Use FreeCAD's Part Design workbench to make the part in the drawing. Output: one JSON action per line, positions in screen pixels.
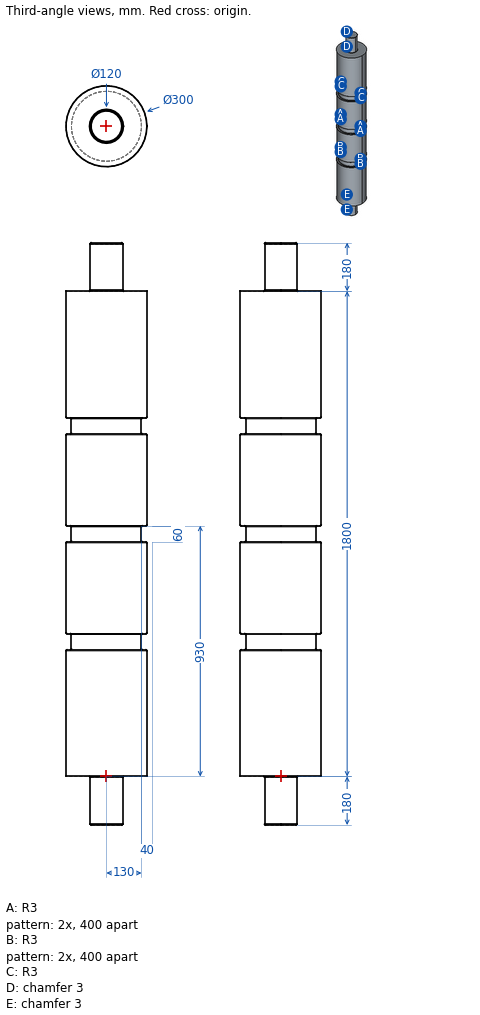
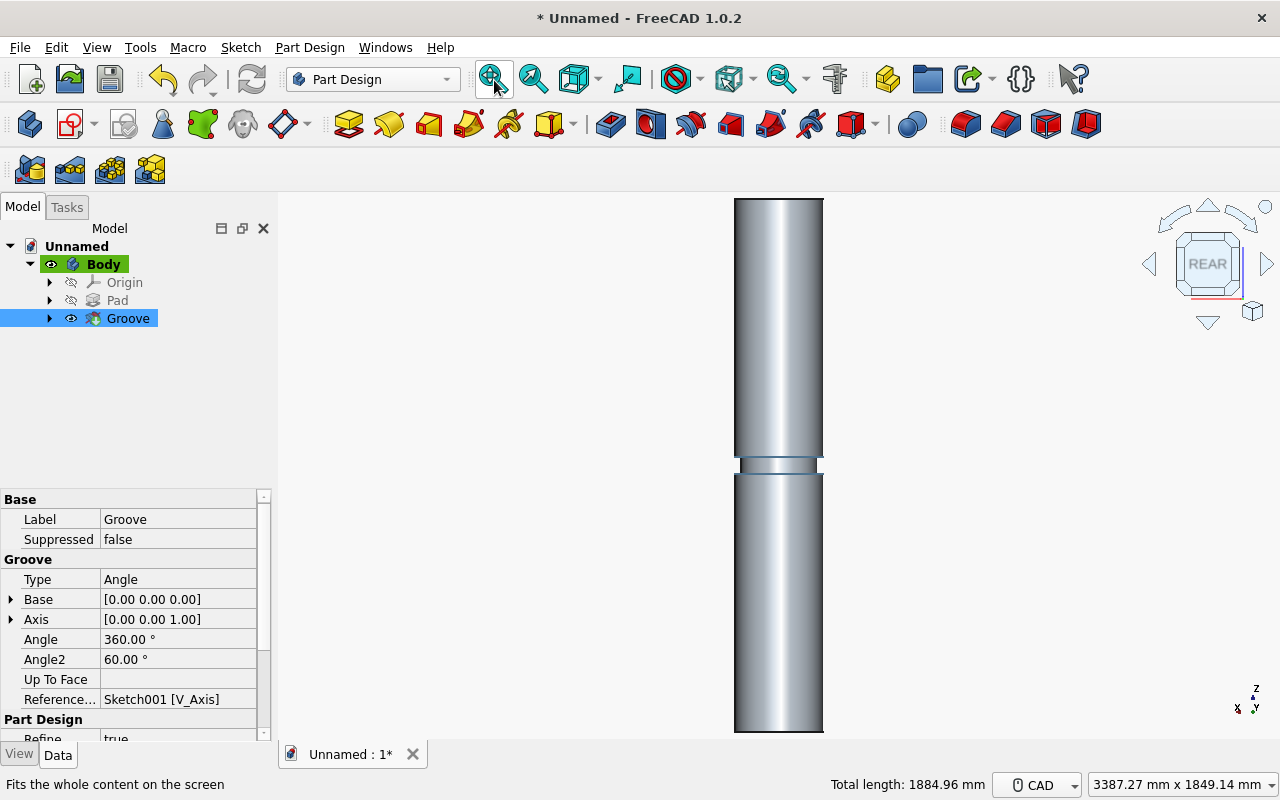
{"action": "key", "text": "6"}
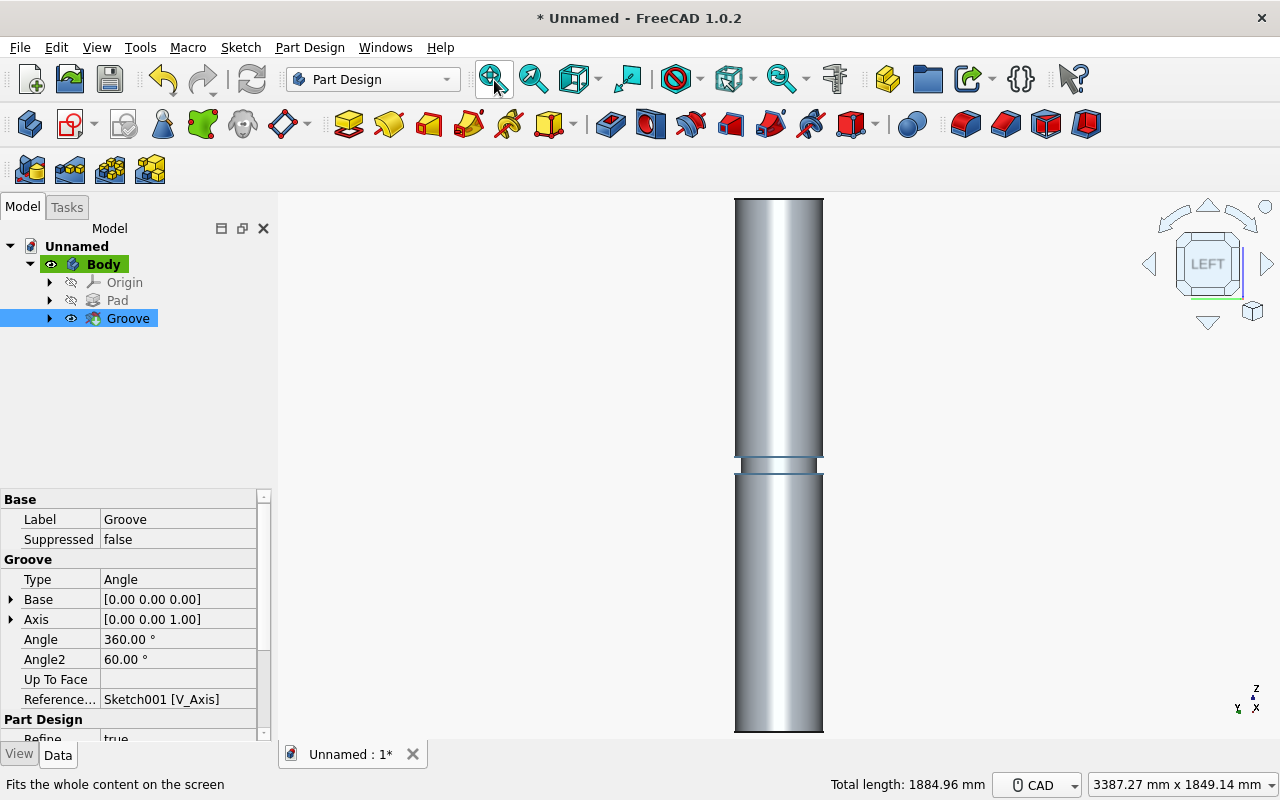
{"action": "key", "text": "v 3"}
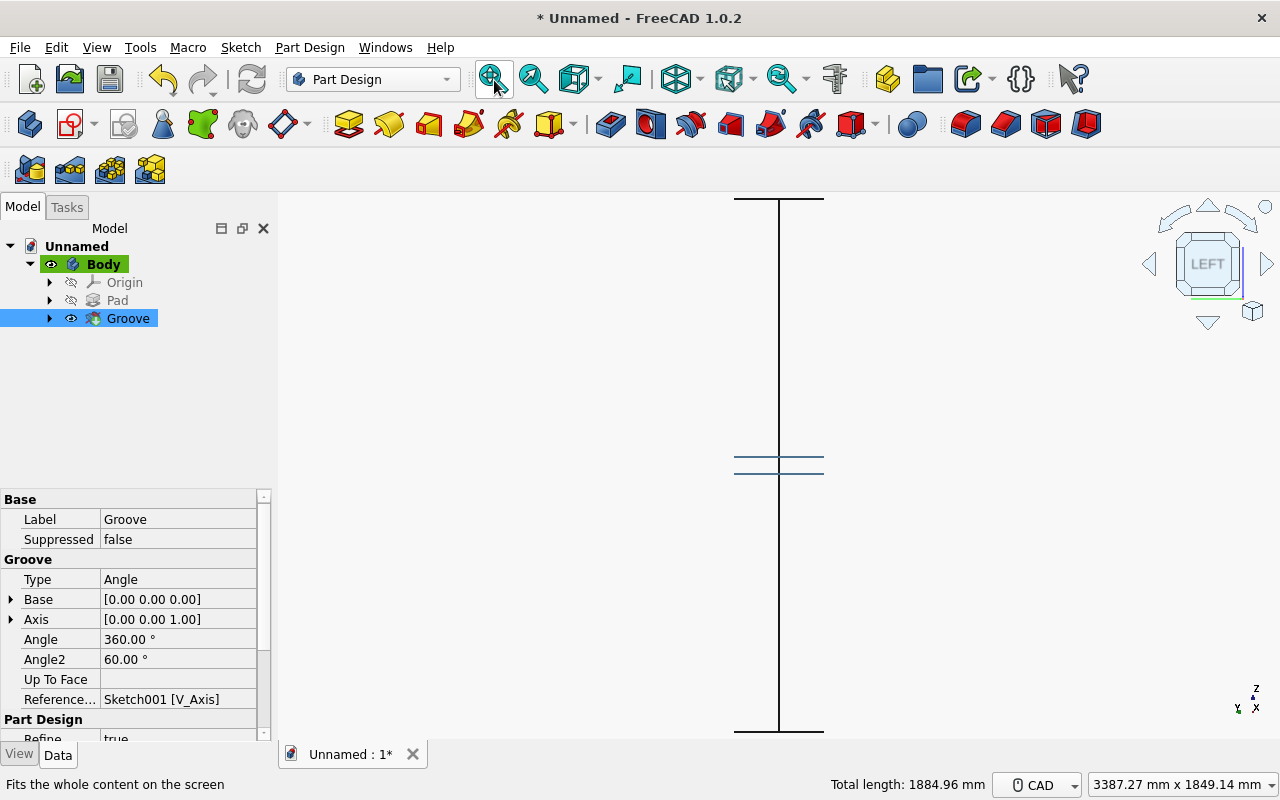
{"action": "key", "text": "0"}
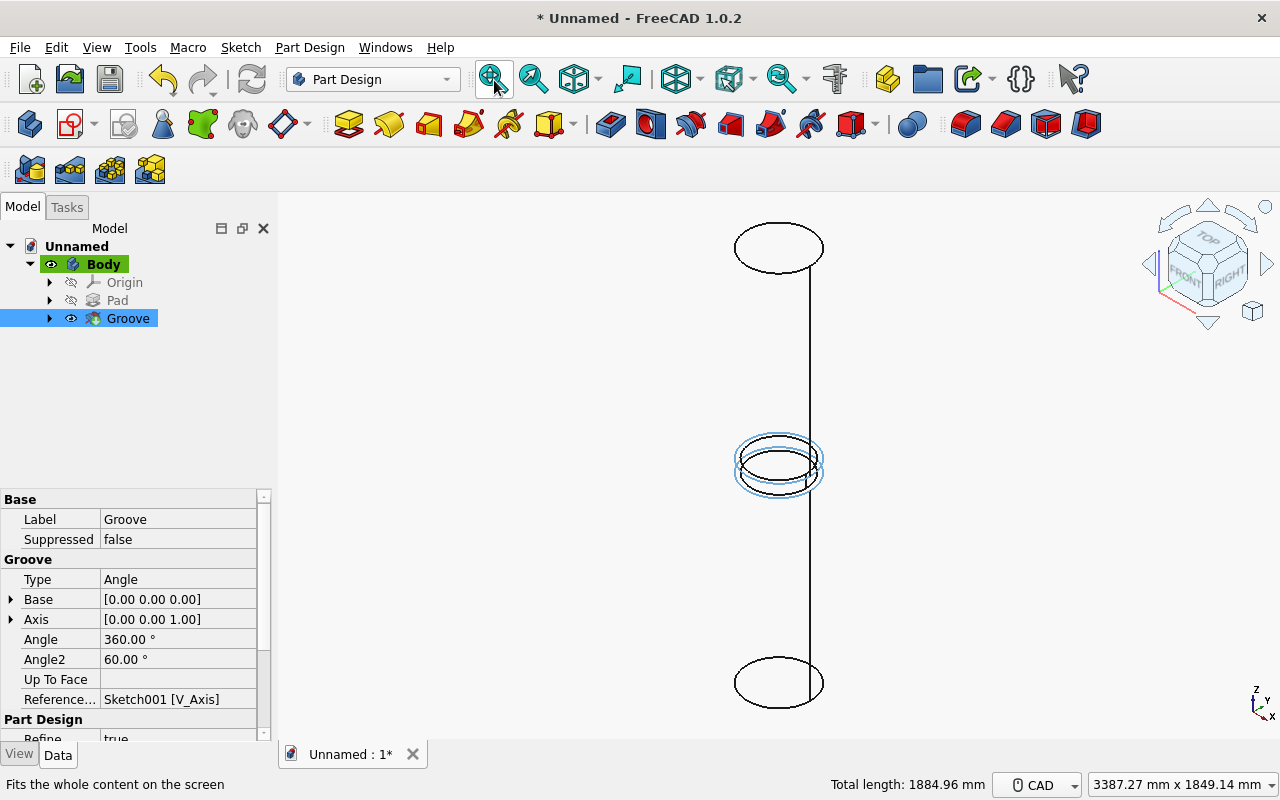
{"action": "left_click", "coordinate": [752, 442], "text": "ctrl"}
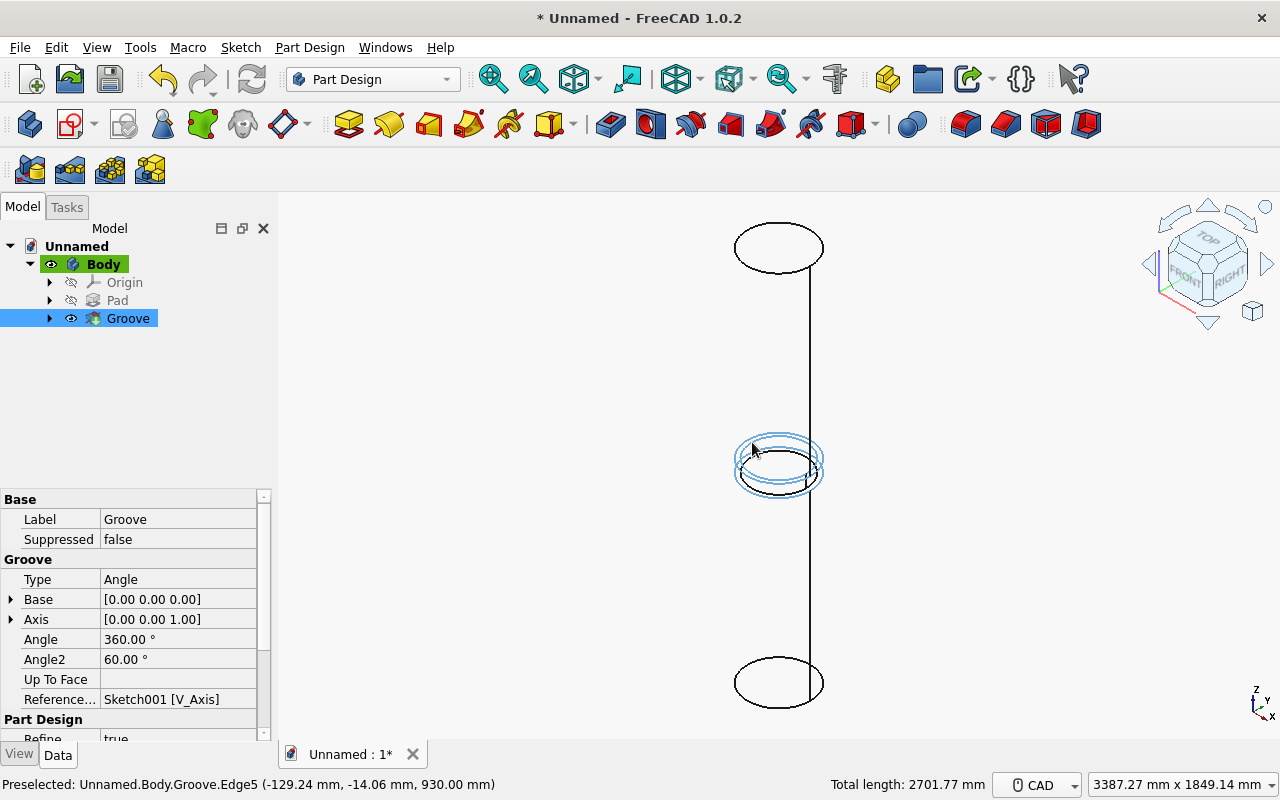
{"action": "left_click", "coordinate": [752, 456], "text": "ctrl"}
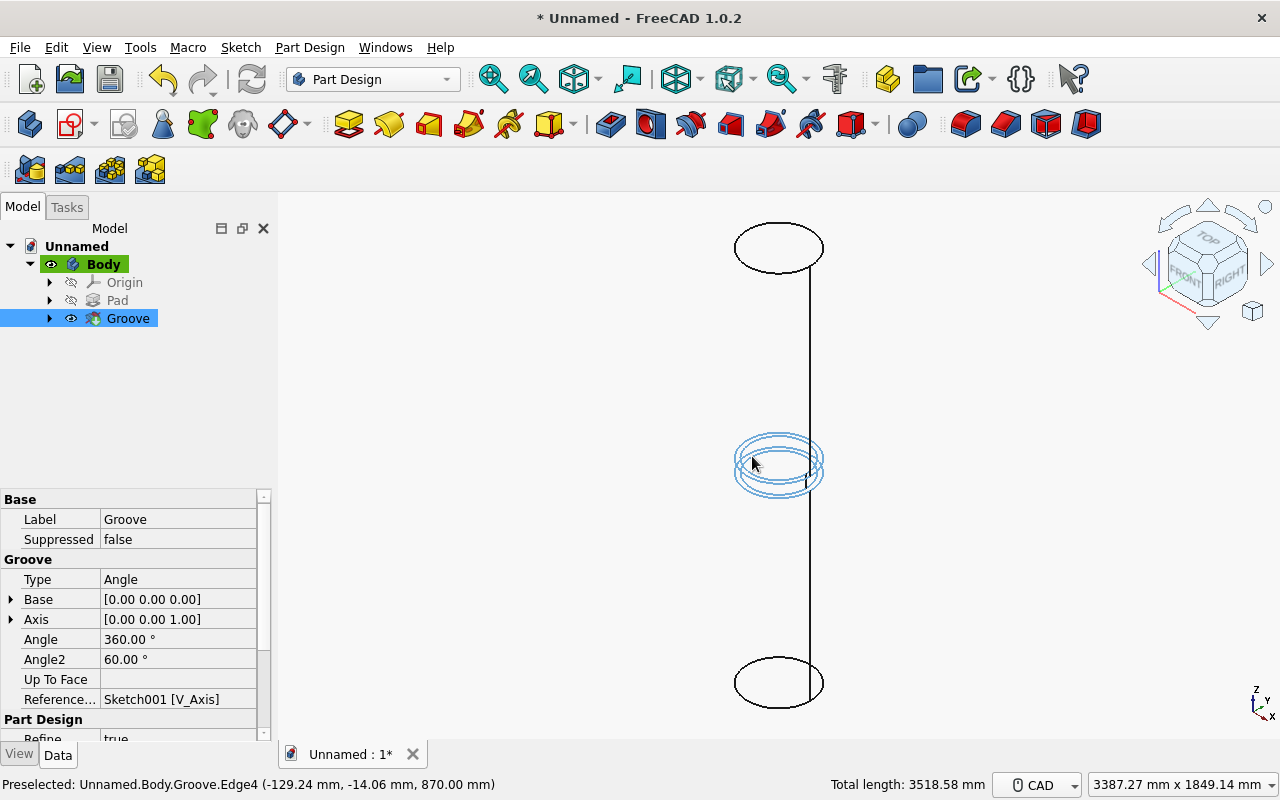
{"action": "key", "text": "v 1"}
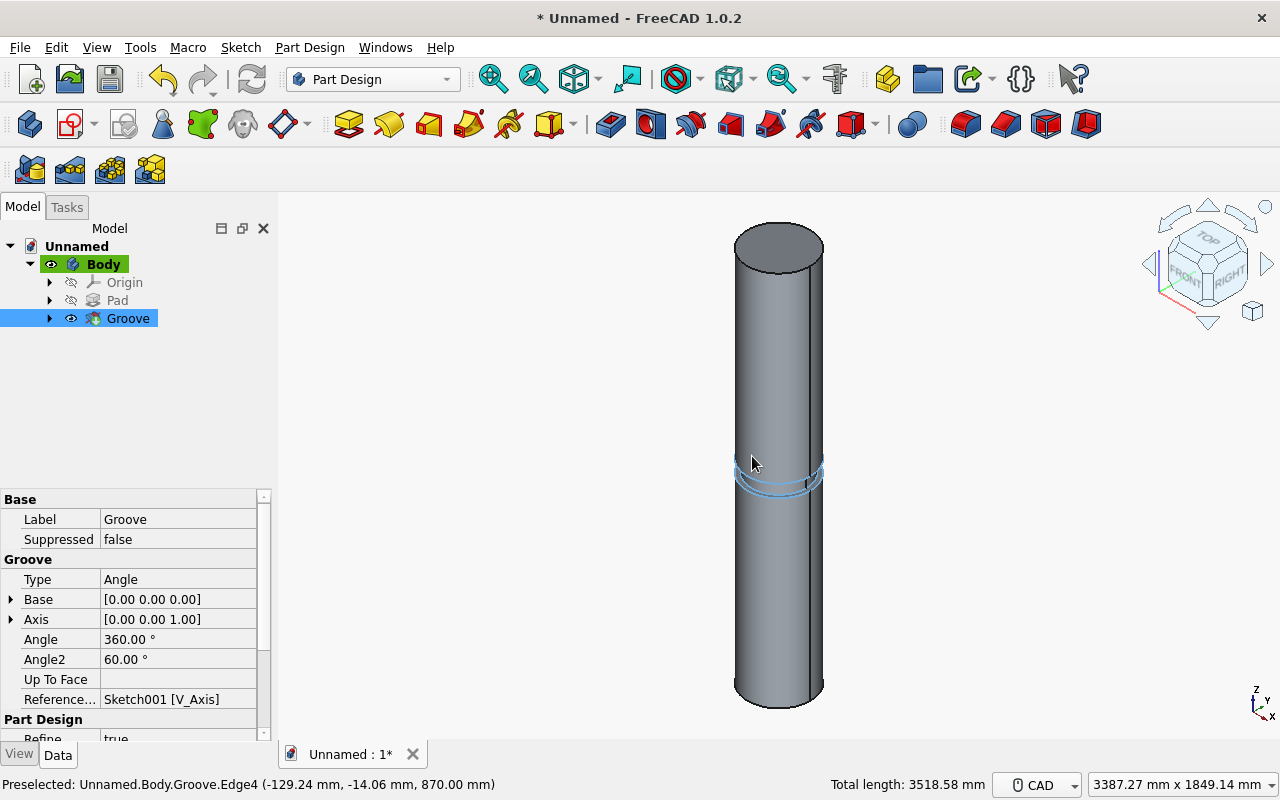
{"action": "left_click", "coordinate": [966, 124]}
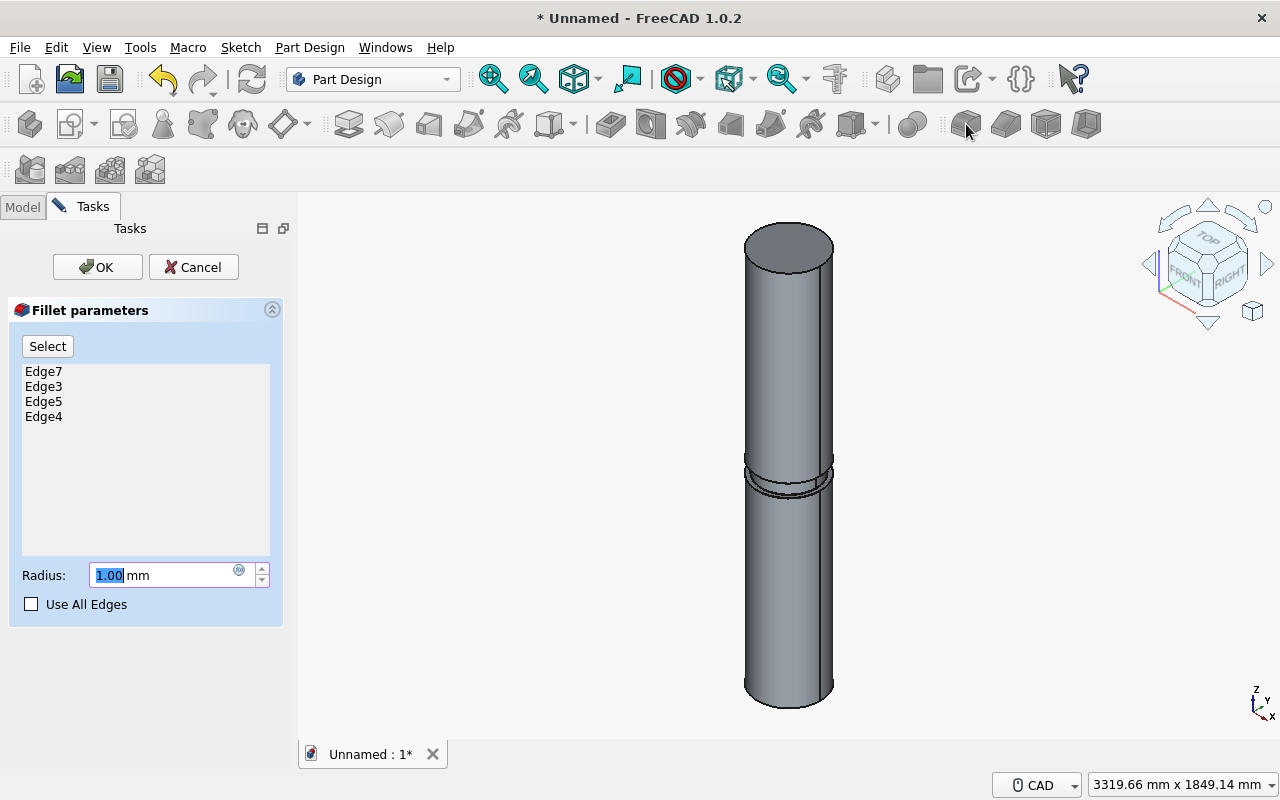
{"action": "type", "text": "3"}
{"action": "key", "text": "Tab"}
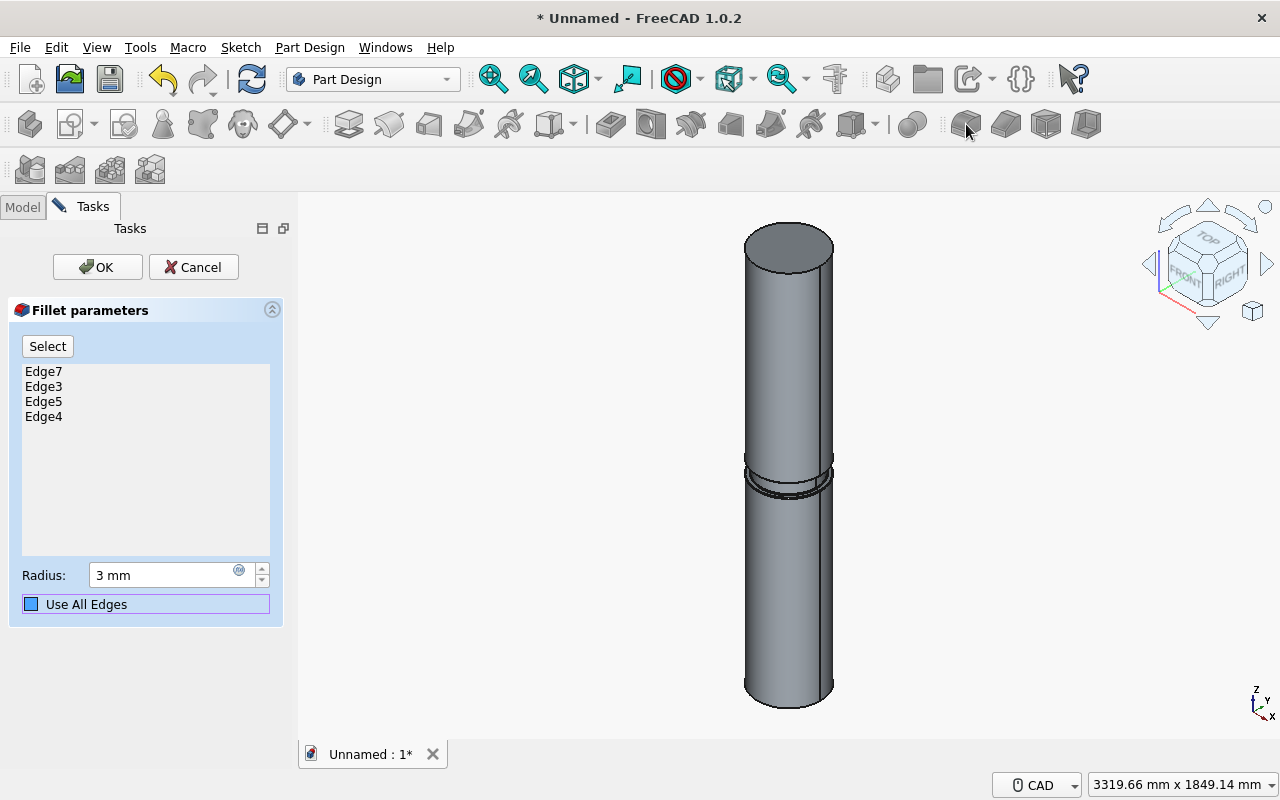
{"action": "left_click", "coordinate": [98, 267]}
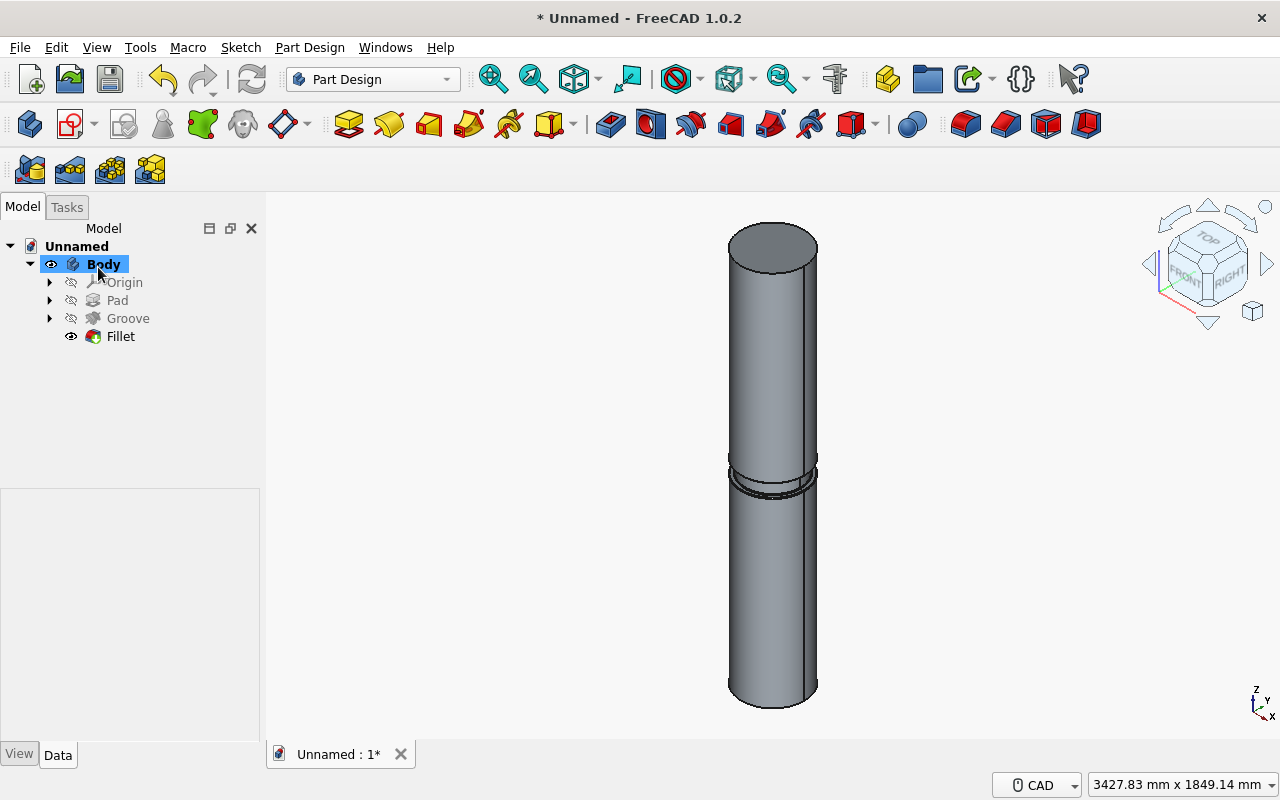
{"action": "left_click", "coordinate": [116, 318]}